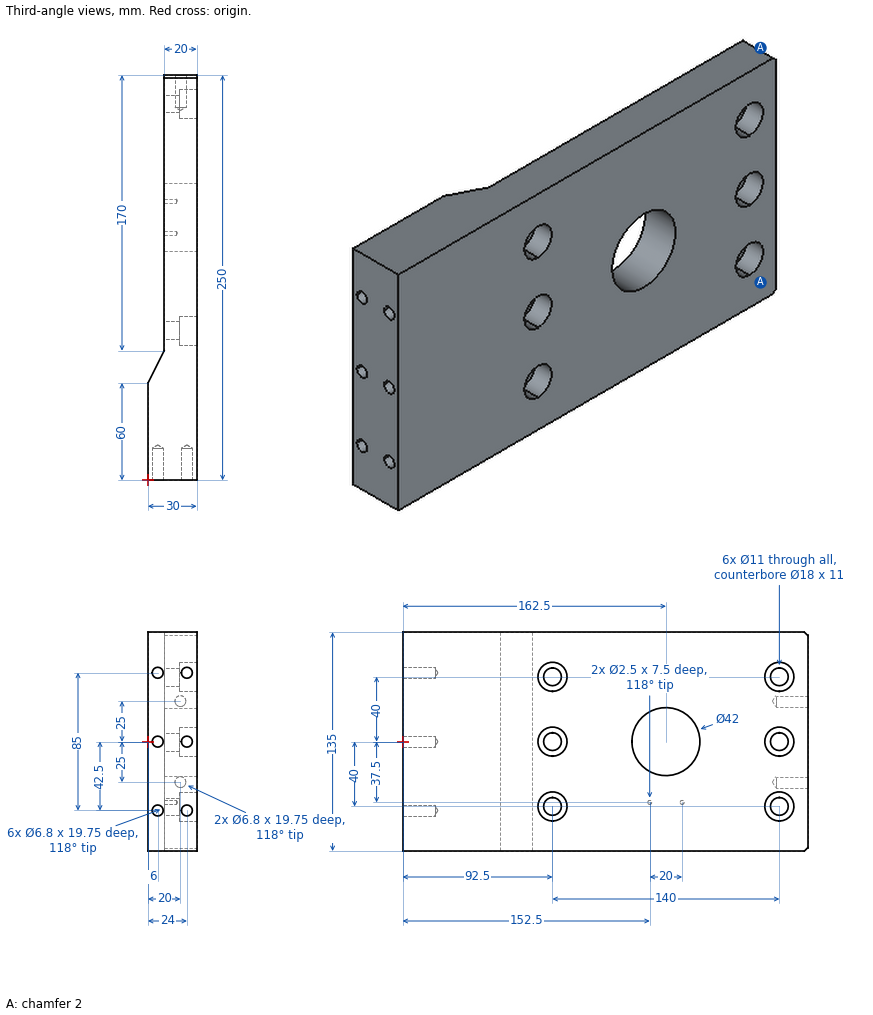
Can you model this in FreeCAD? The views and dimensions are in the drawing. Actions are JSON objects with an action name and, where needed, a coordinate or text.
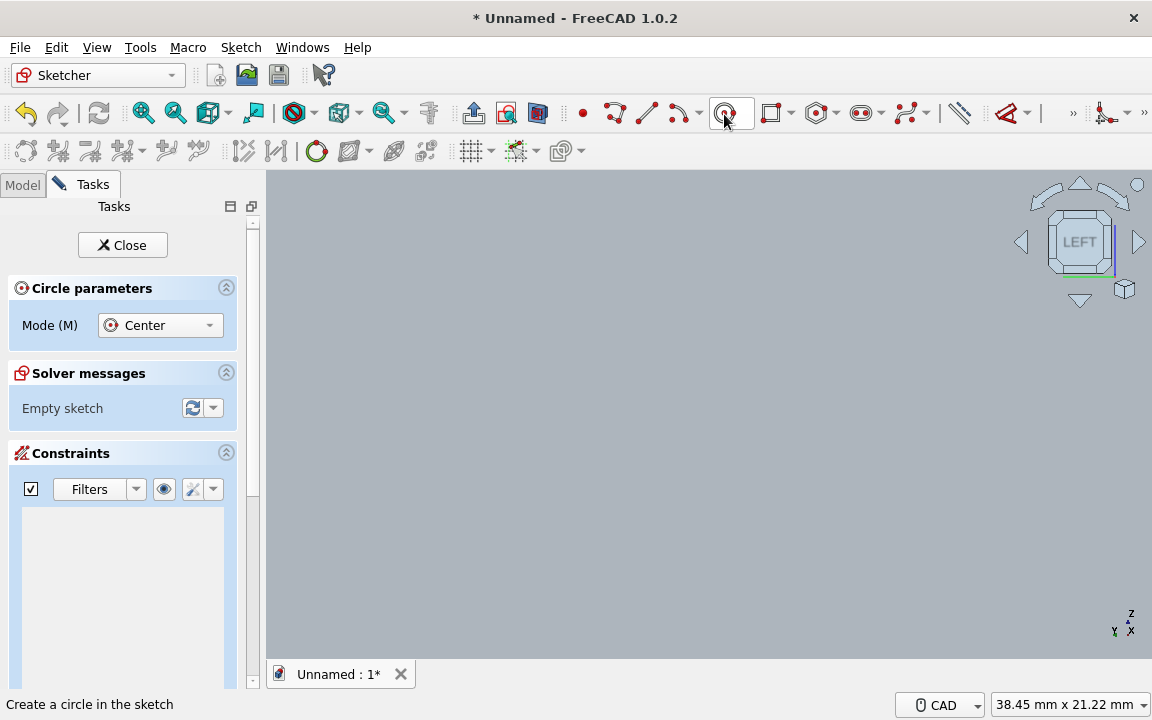
{"action": "left_click", "coordinate": [868, 404]}
{"action": "mouse_move", "coordinate": [888, 384]}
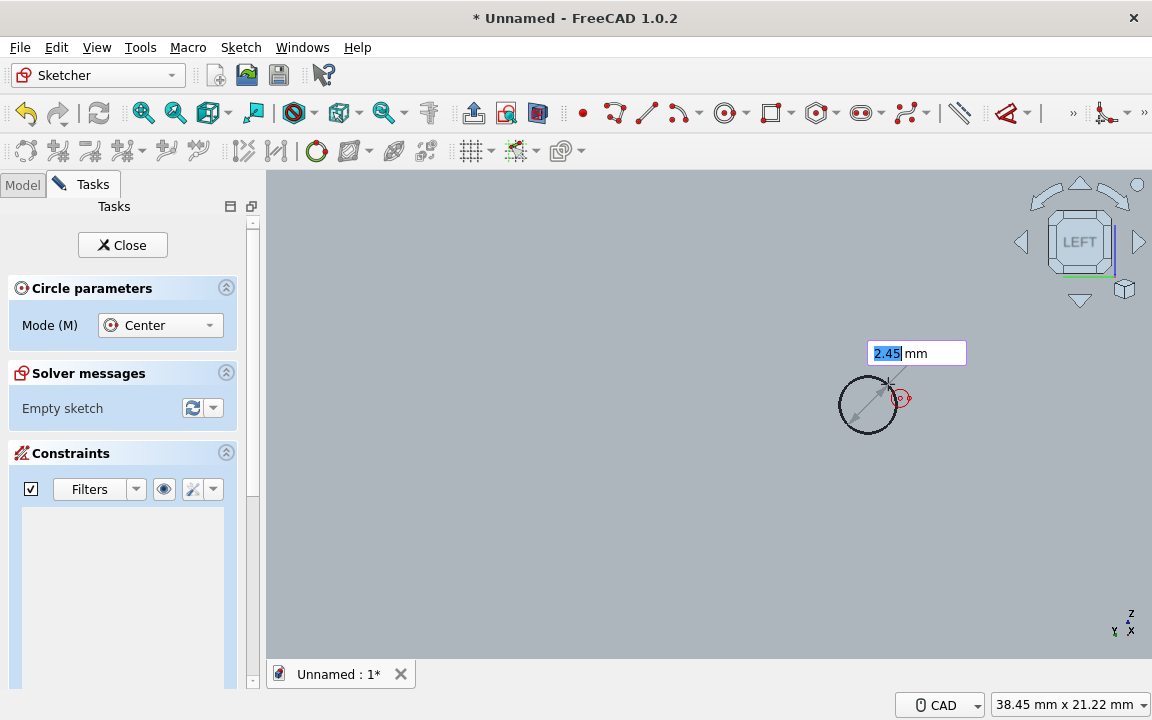
{"action": "type", "text": "2.5"}
{"action": "key", "text": "Return"}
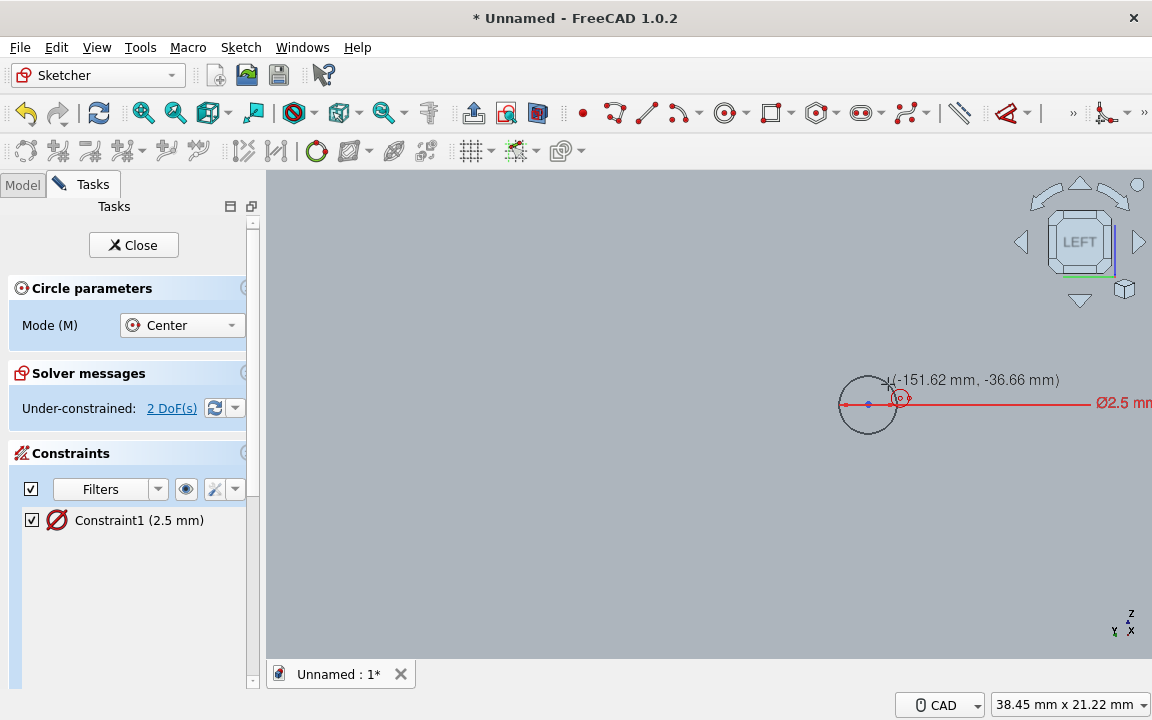
{"action": "left_click", "coordinate": [407, 404]}
{"action": "mouse_move", "coordinate": [427, 384]}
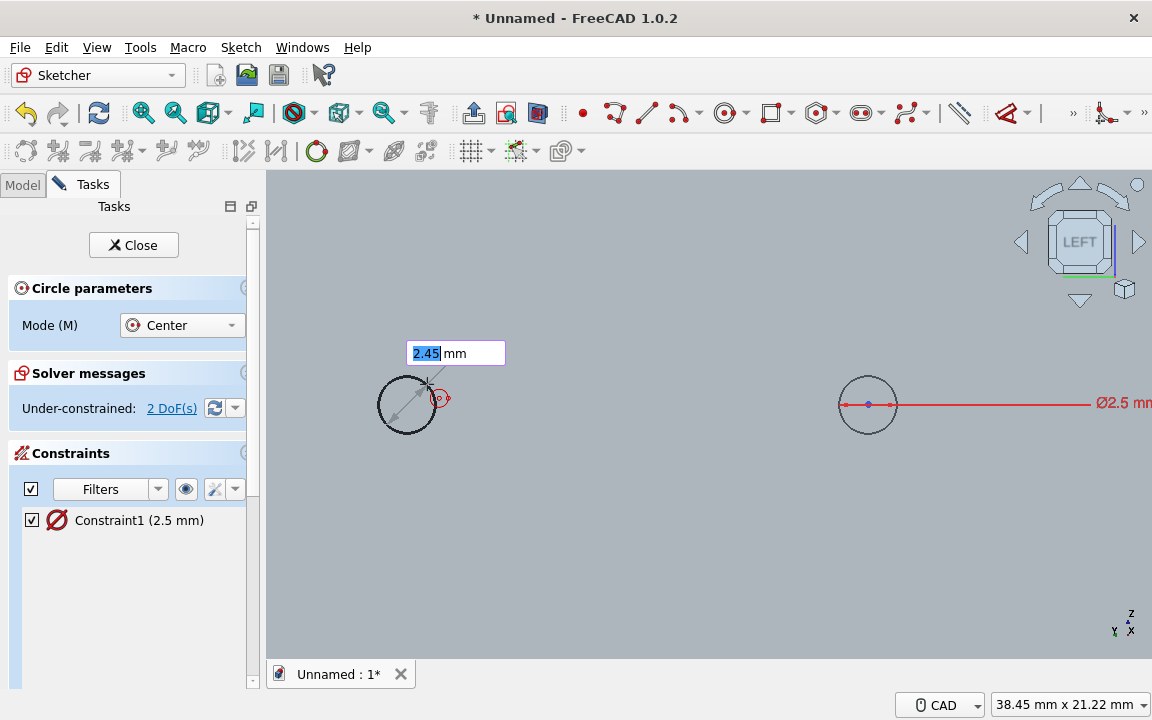
{"action": "type", "text": "2.5"}
{"action": "key", "text": "Return"}
{"action": "key", "text": "Escape"}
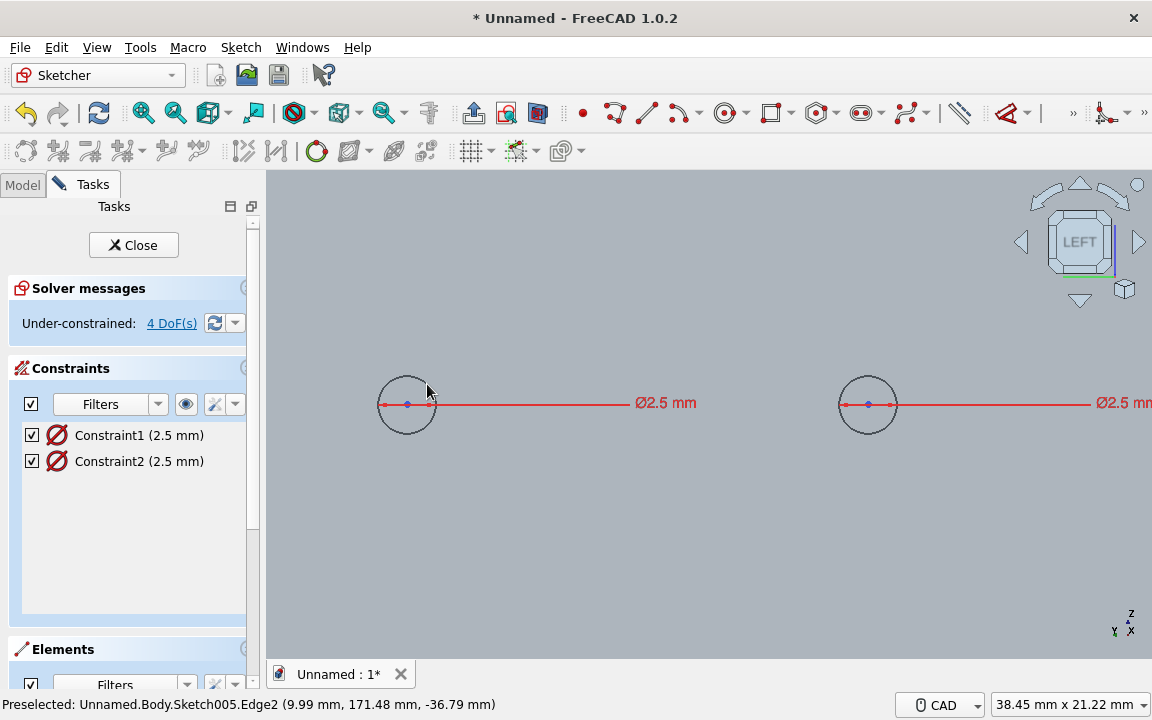
{"action": "left_click", "coordinate": [868, 405]}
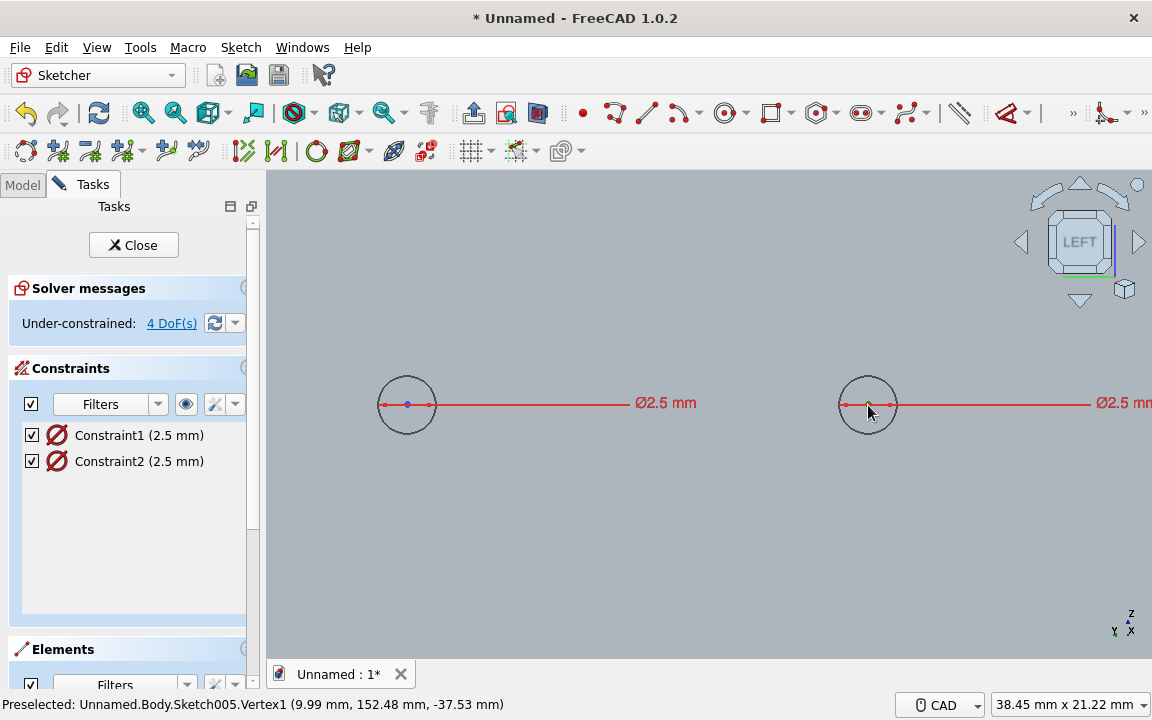
{"action": "left_click", "coordinate": [407, 405]}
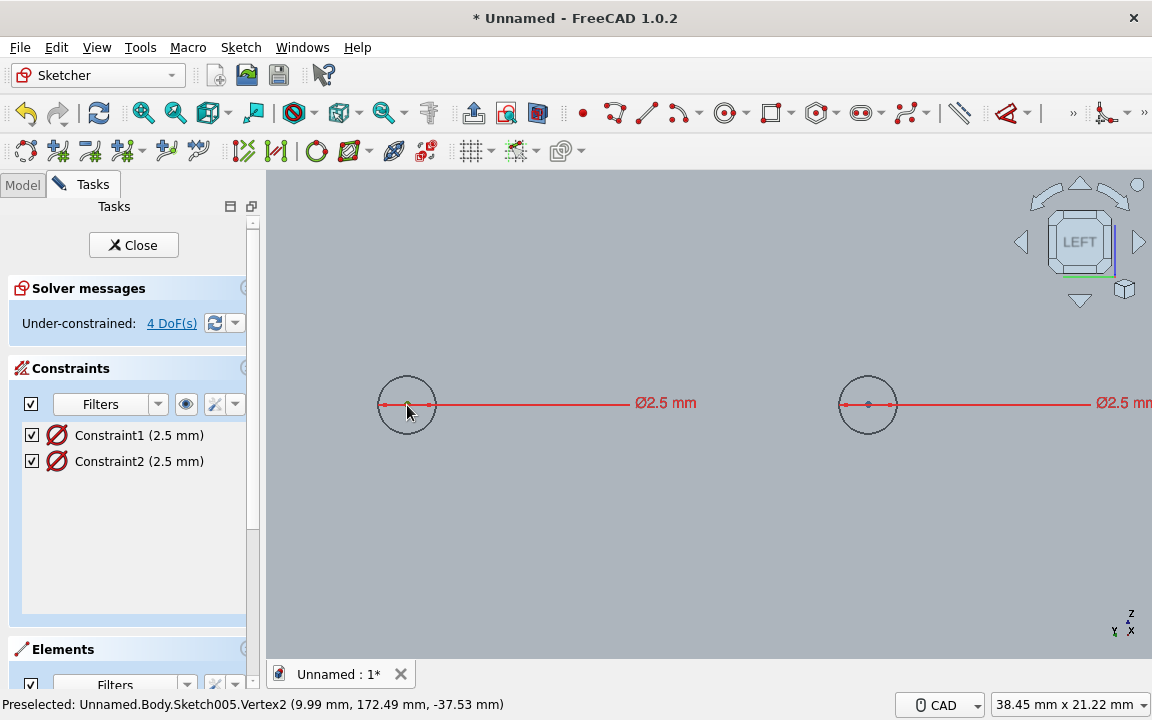
{"action": "key", "text": "h"}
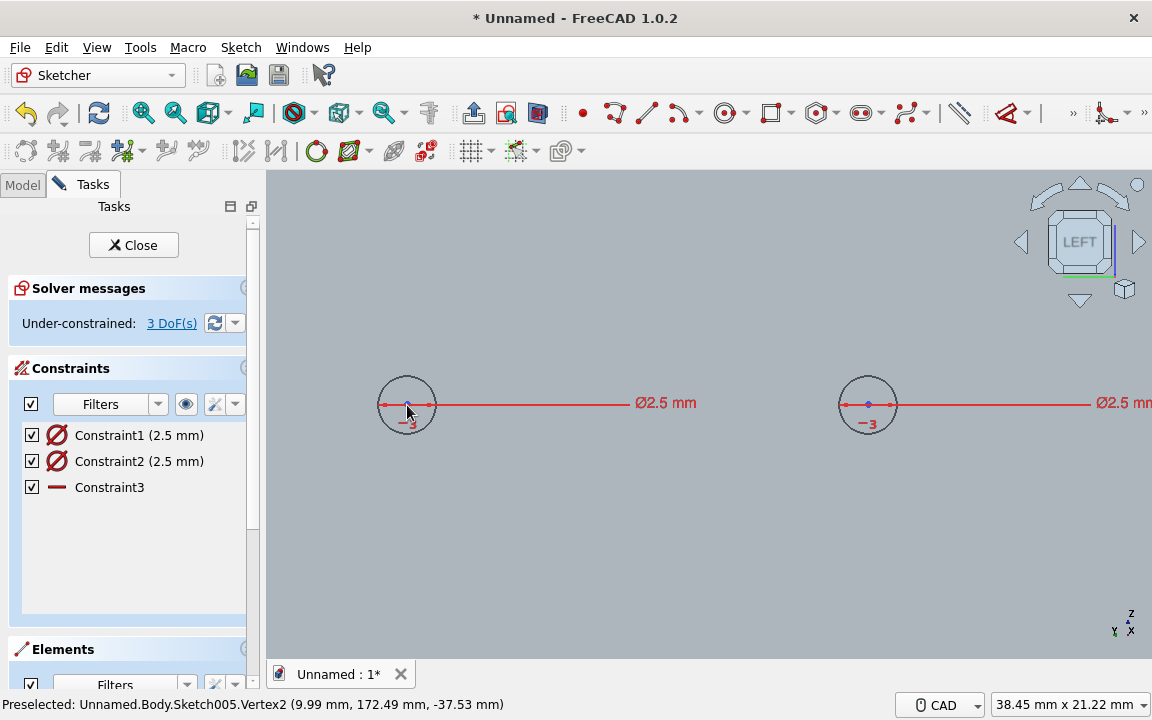
{"action": "left_click", "coordinate": [1006, 114]}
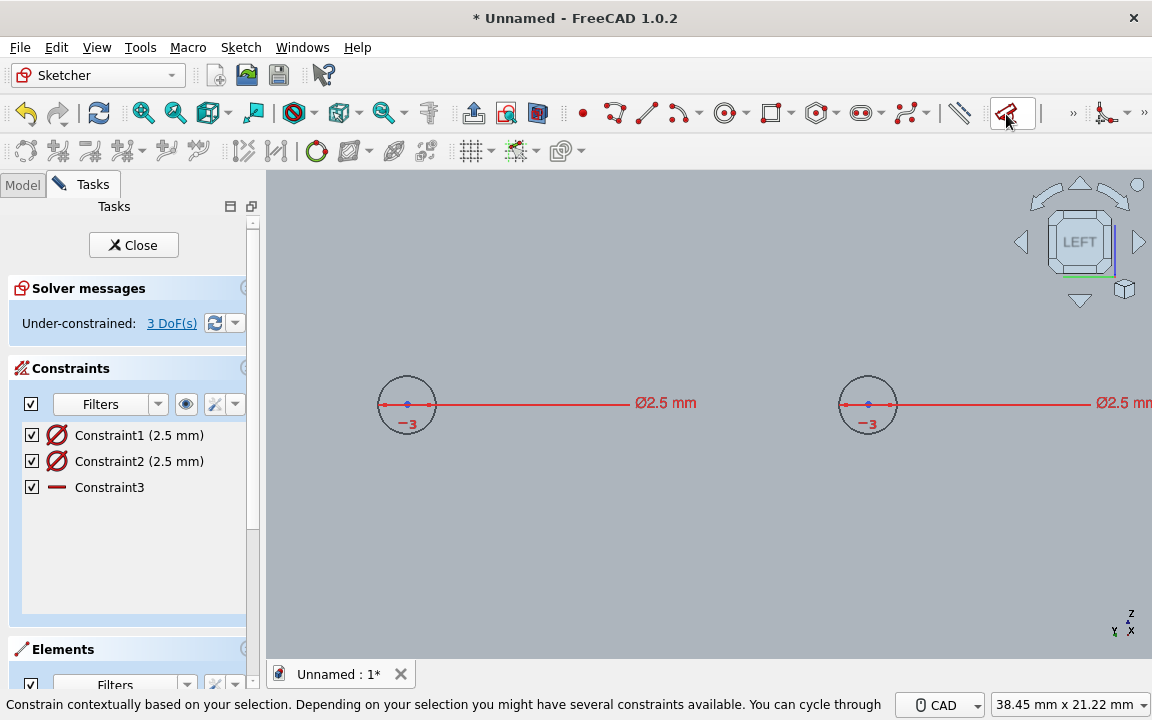
{"action": "left_click", "coordinate": [868, 405]}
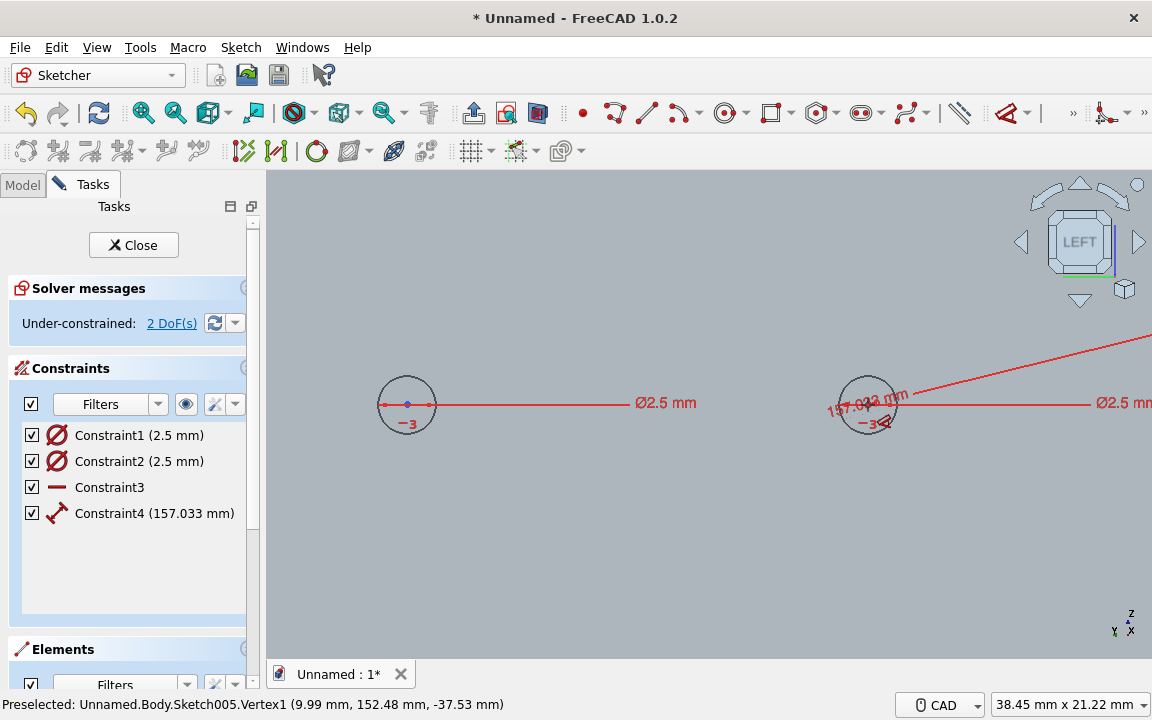
{"action": "left_click", "coordinate": [407, 405]}
{"action": "left_click", "coordinate": [638, 439]}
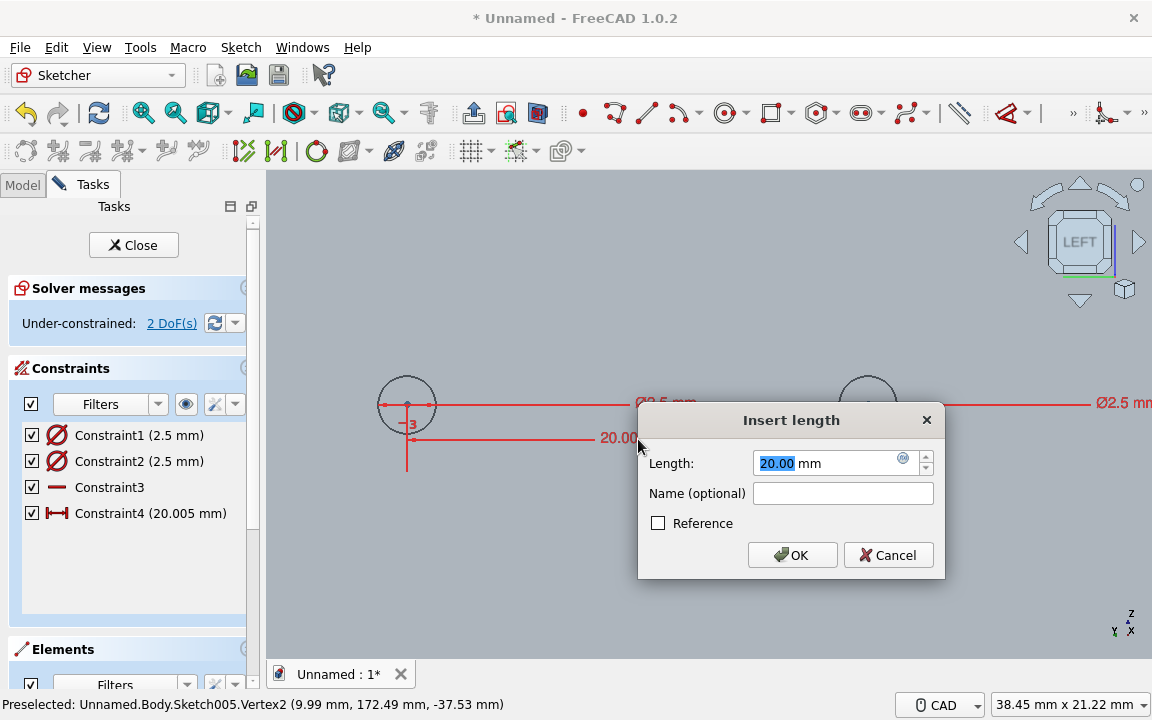
{"action": "type", "text": "20"}
{"action": "key", "text": "Return"}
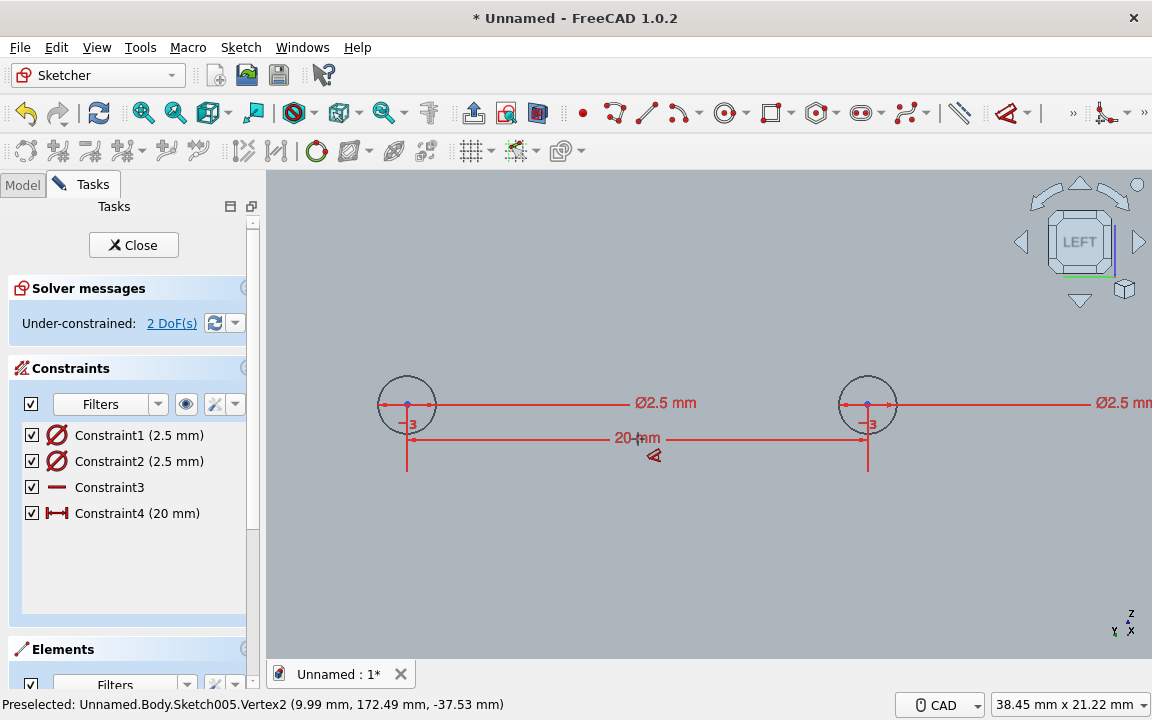
{"action": "left_click", "coordinate": [868, 405]}
{"action": "left_click", "coordinate": [834, 301]}